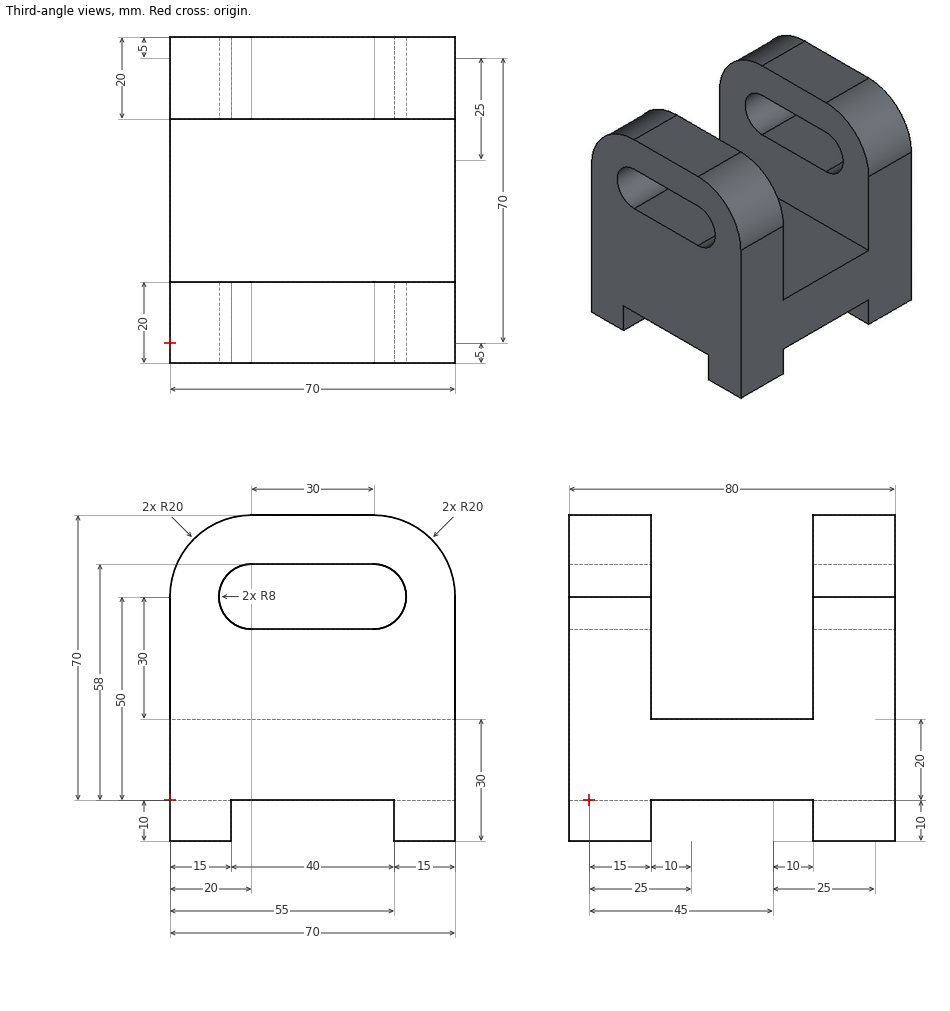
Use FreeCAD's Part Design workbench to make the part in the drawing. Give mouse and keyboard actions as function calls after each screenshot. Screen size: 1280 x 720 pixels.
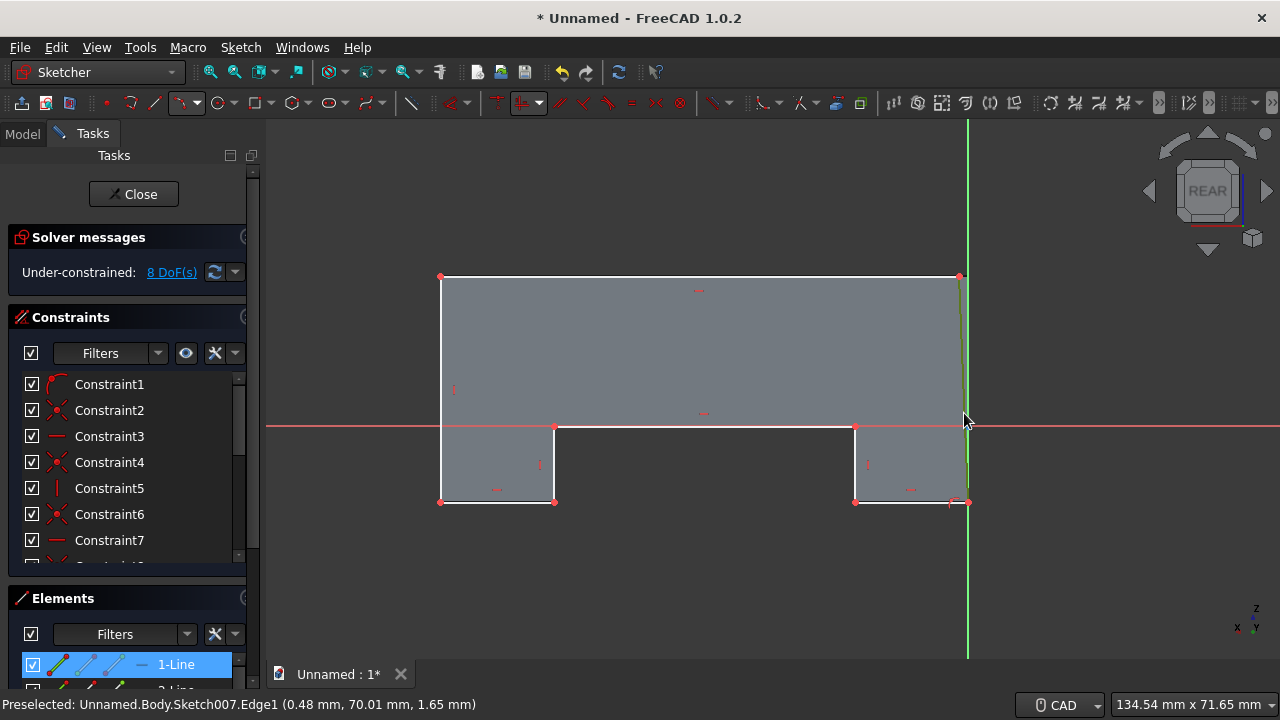
key(v)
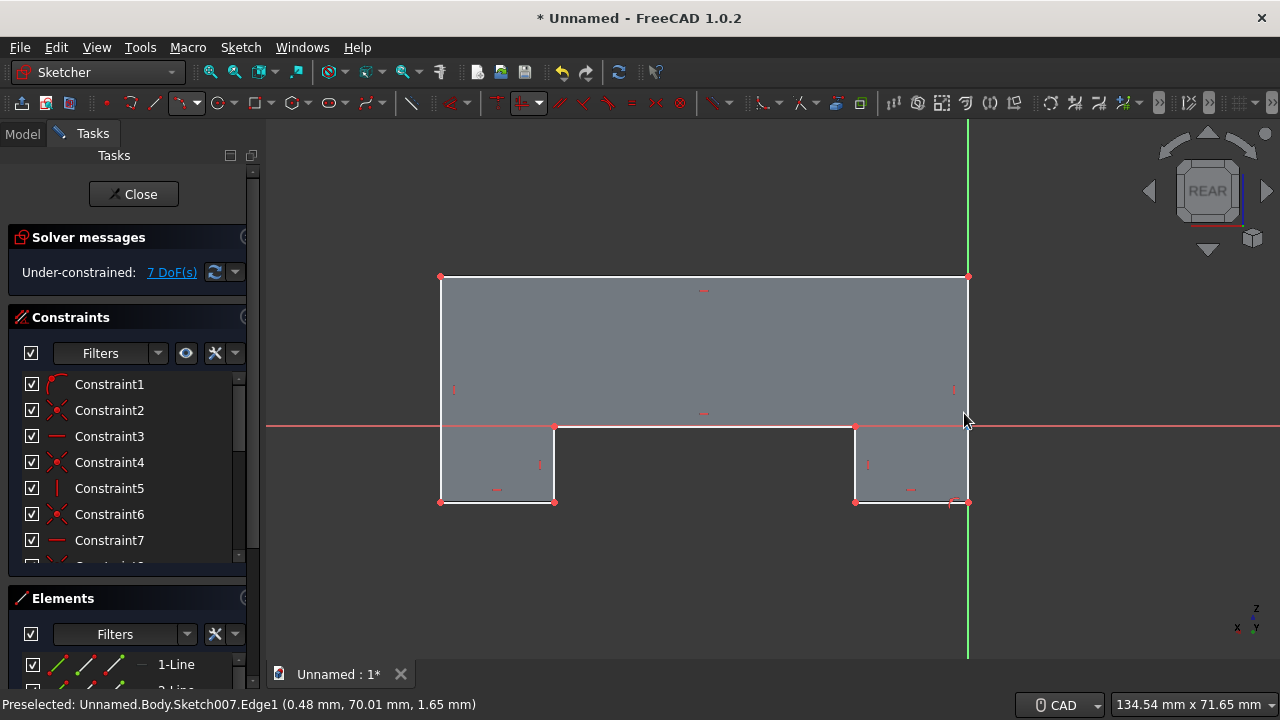
click(554, 427)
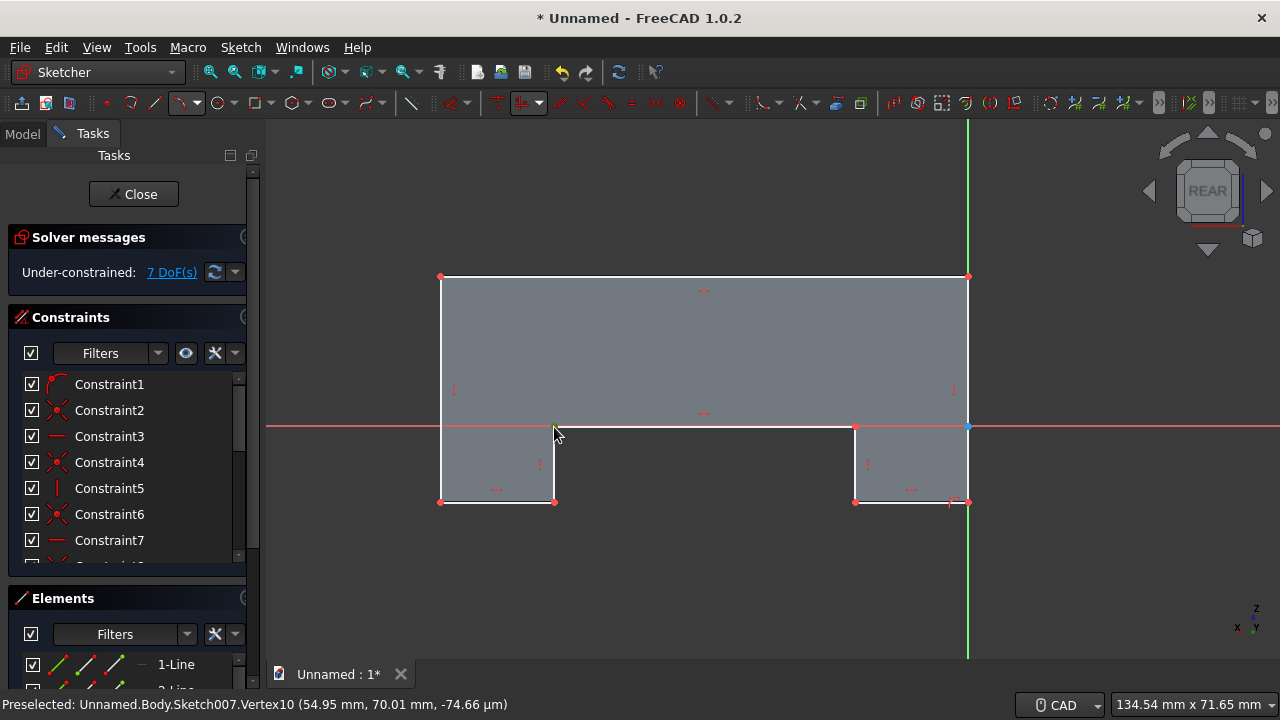
click(353, 426)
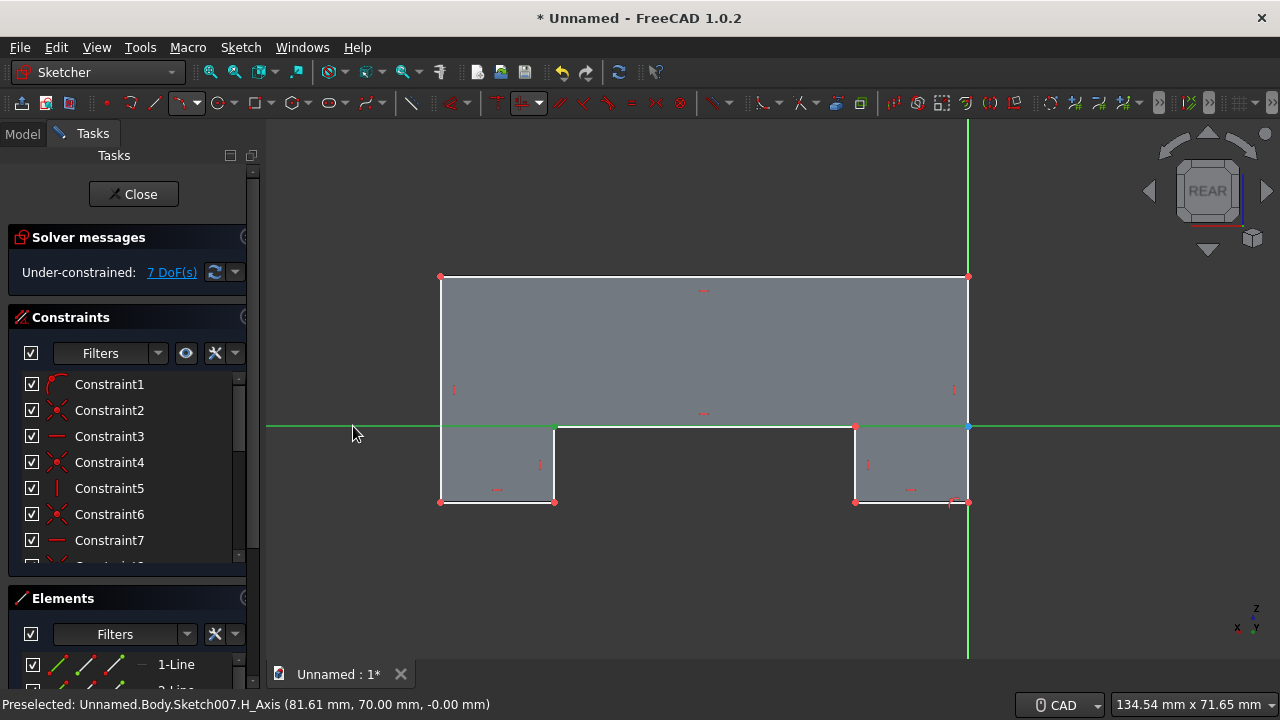
key(c)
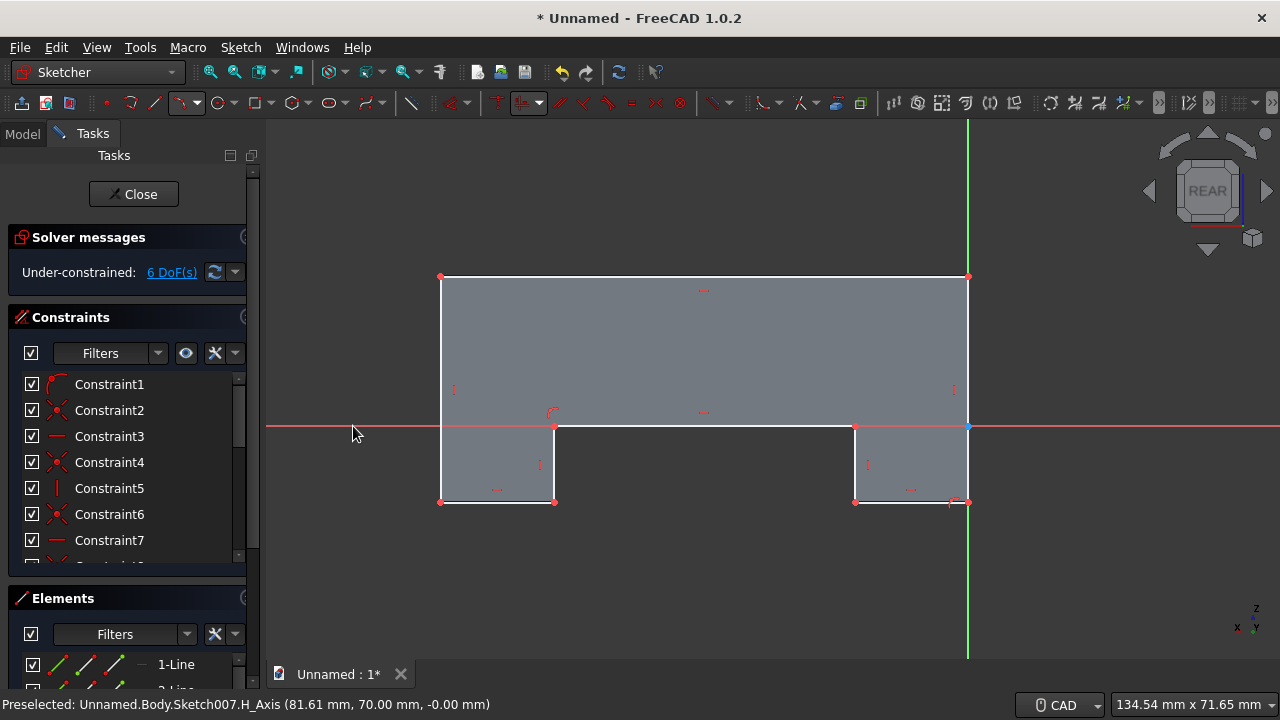
click(450, 104)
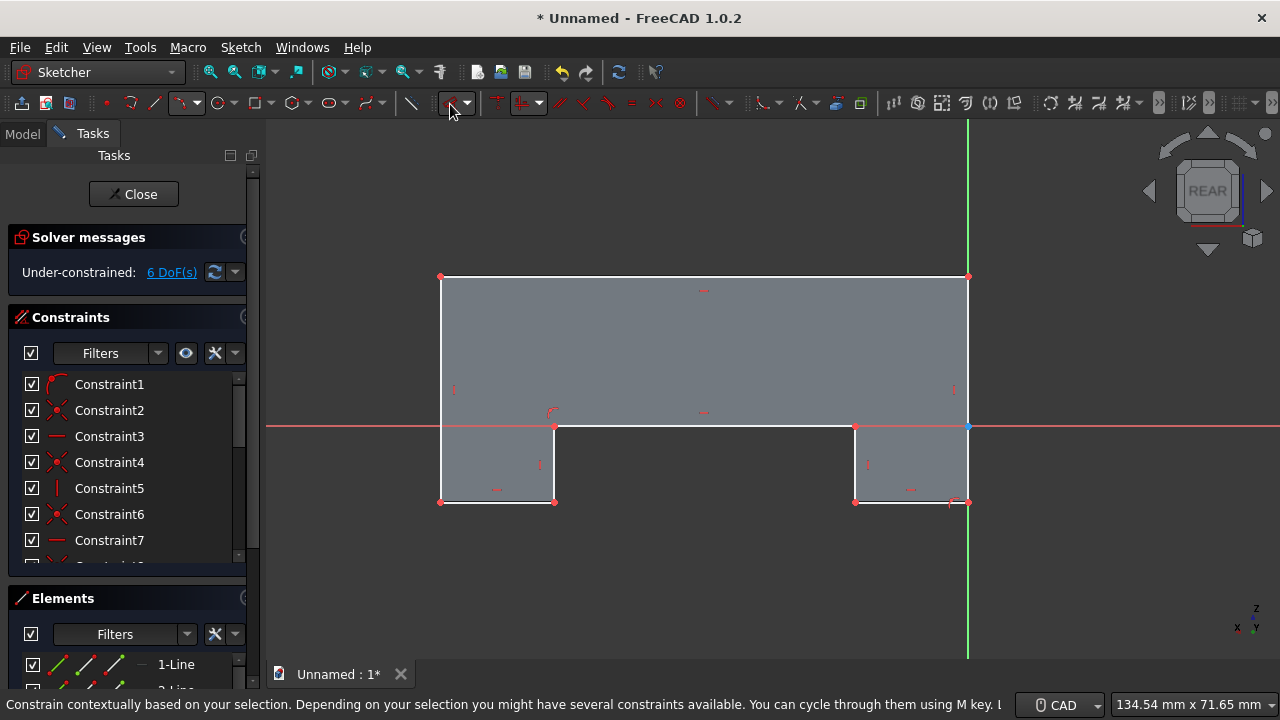
click(968, 345)
click(1002, 390)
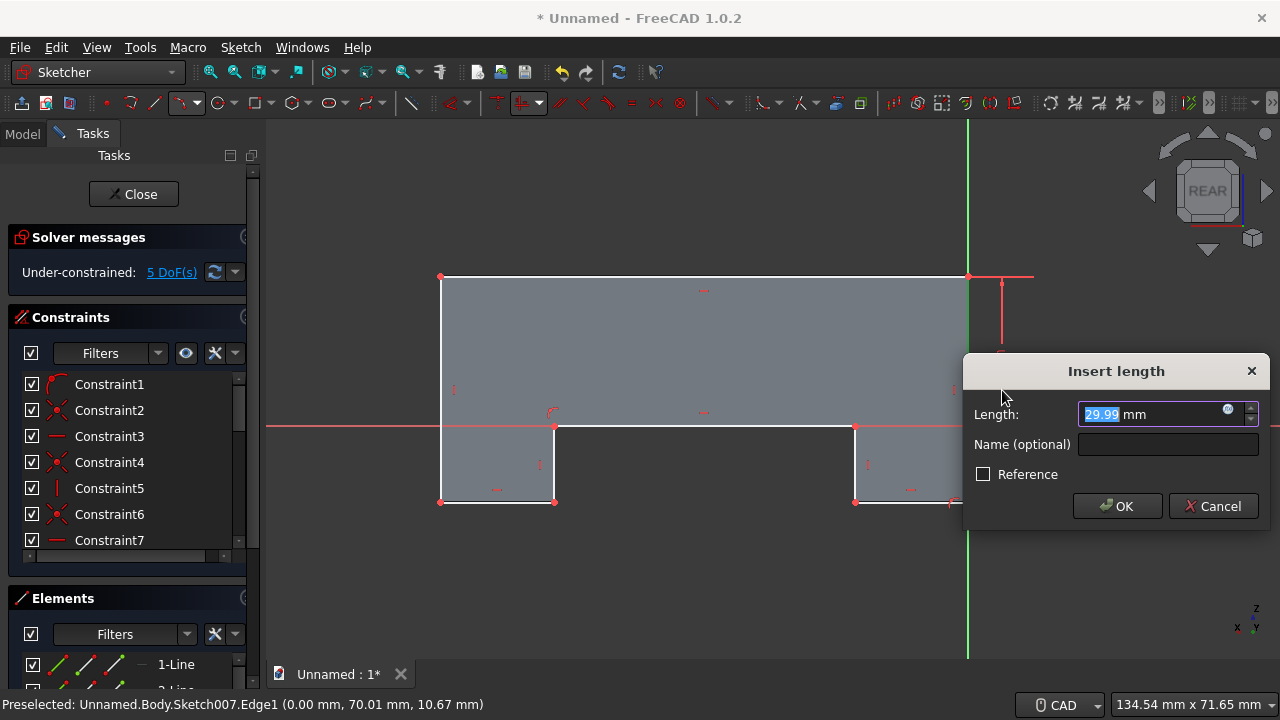
text(30)
key(Return)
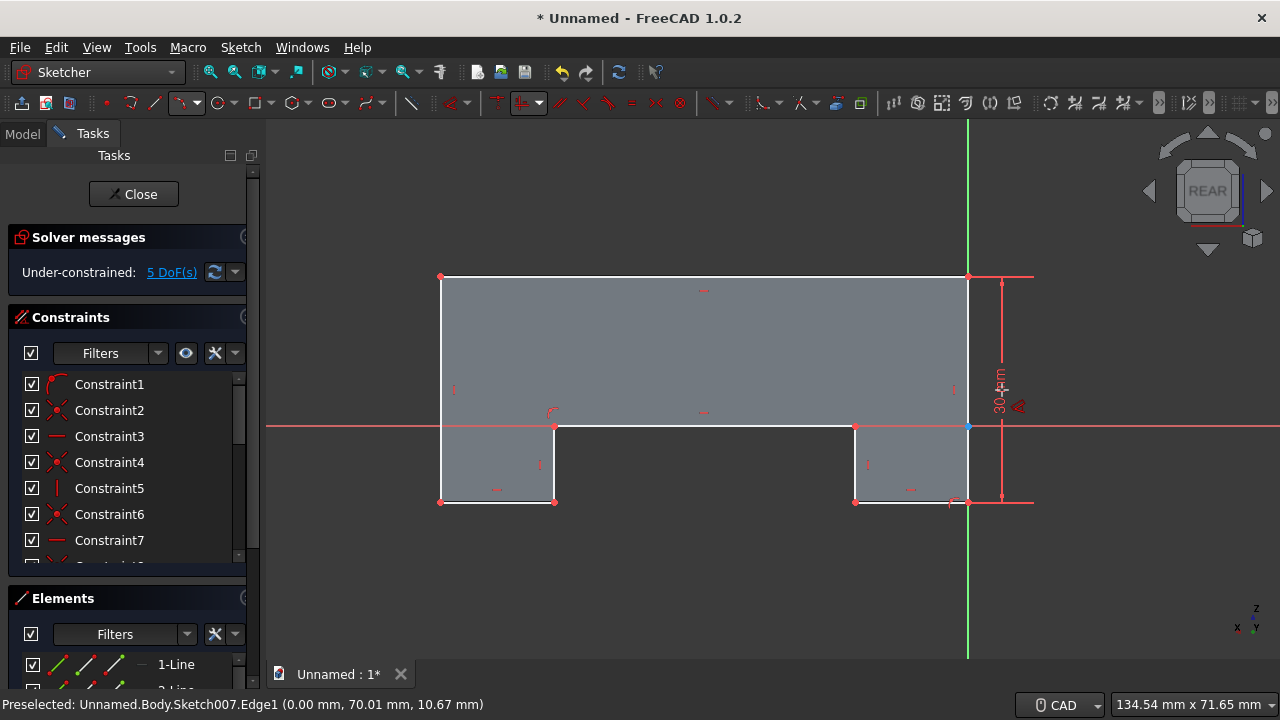
click(810, 277)
click(705, 243)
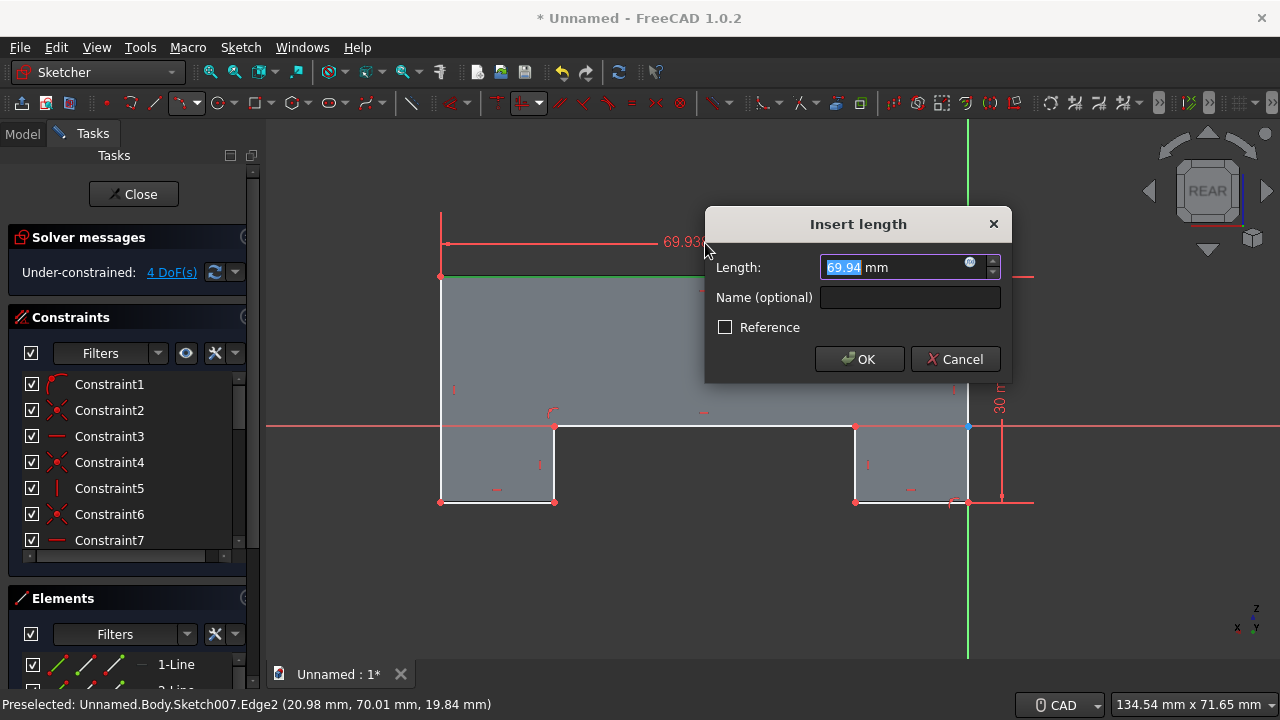
text(70)
key(Return)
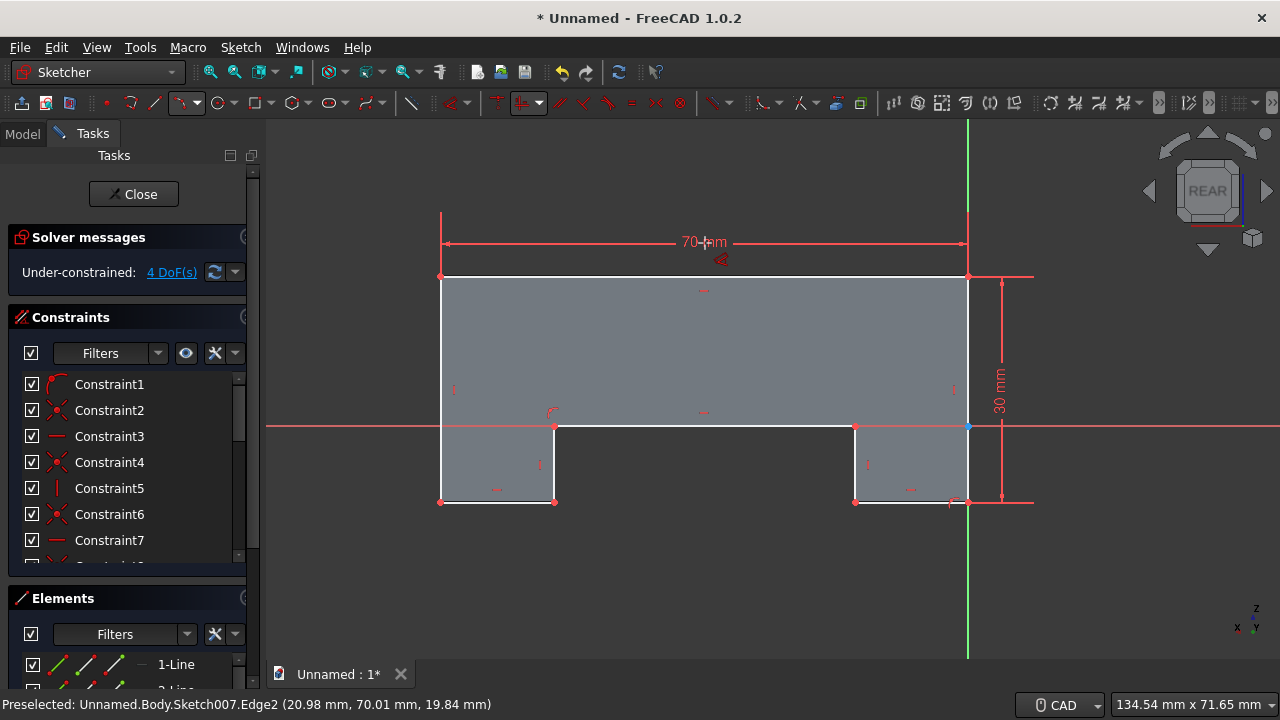
click(441, 345)
click(407, 390)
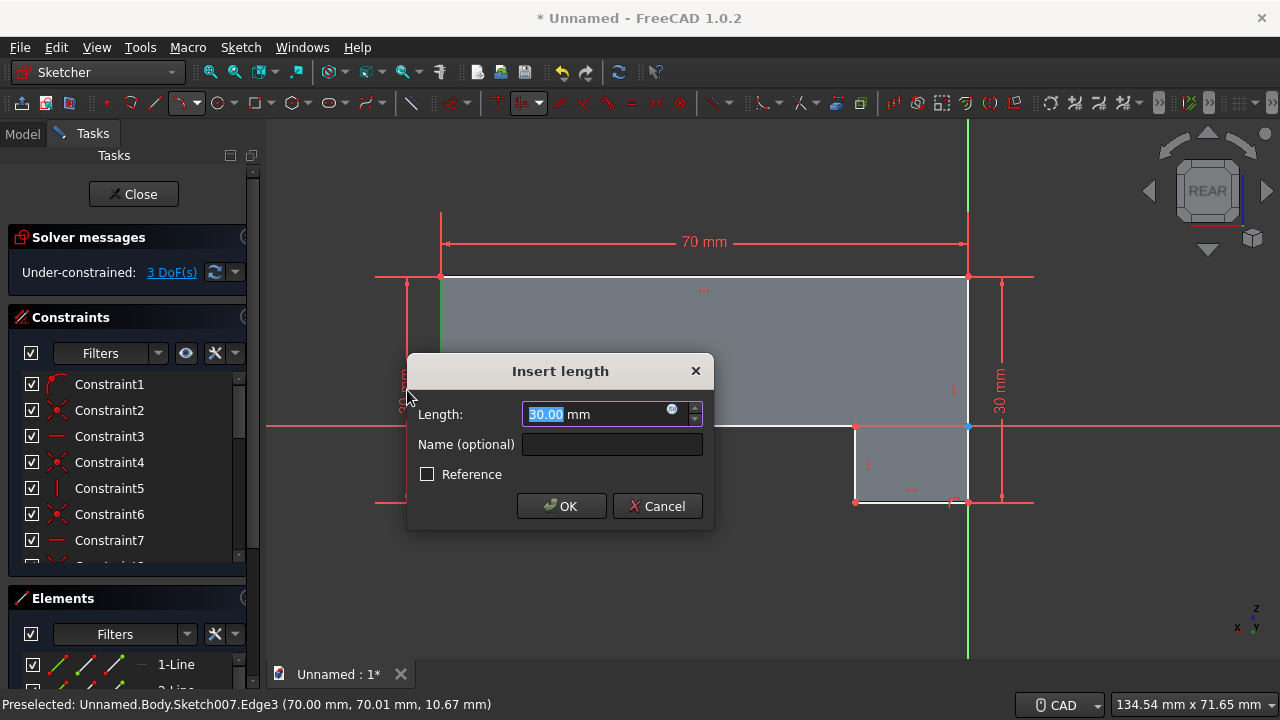
text(30)
key(Return)